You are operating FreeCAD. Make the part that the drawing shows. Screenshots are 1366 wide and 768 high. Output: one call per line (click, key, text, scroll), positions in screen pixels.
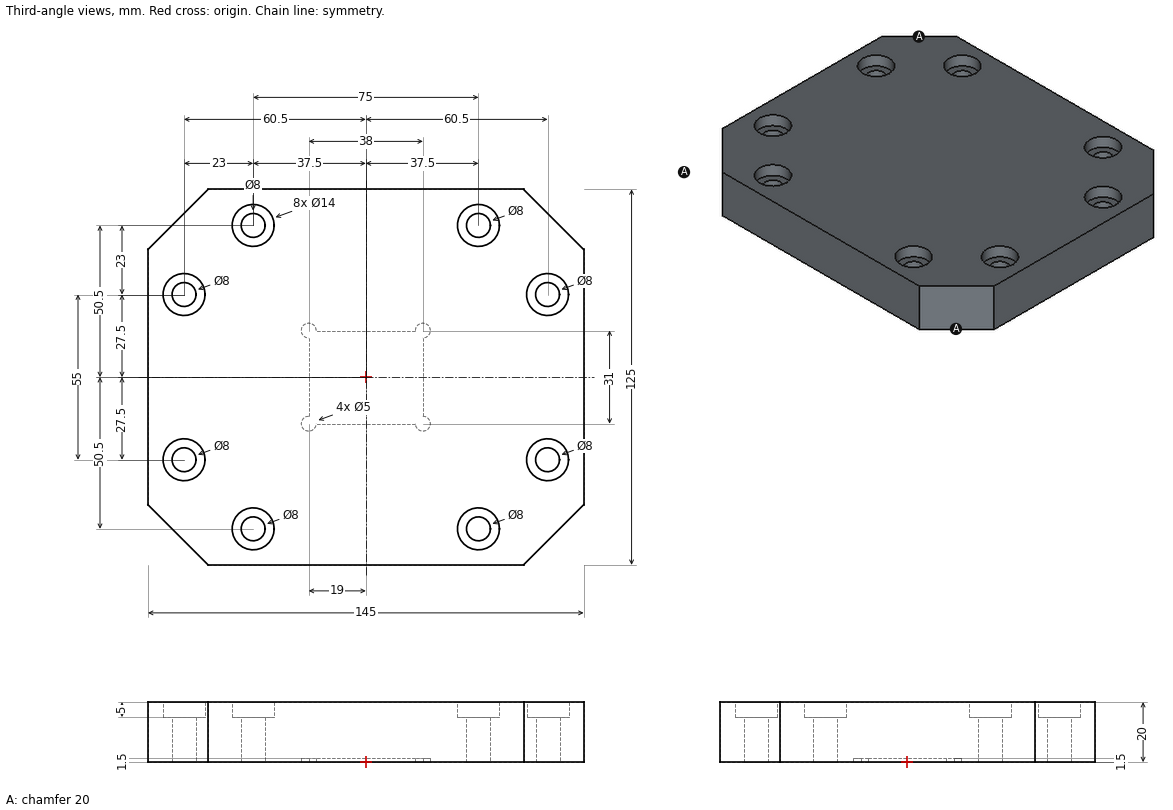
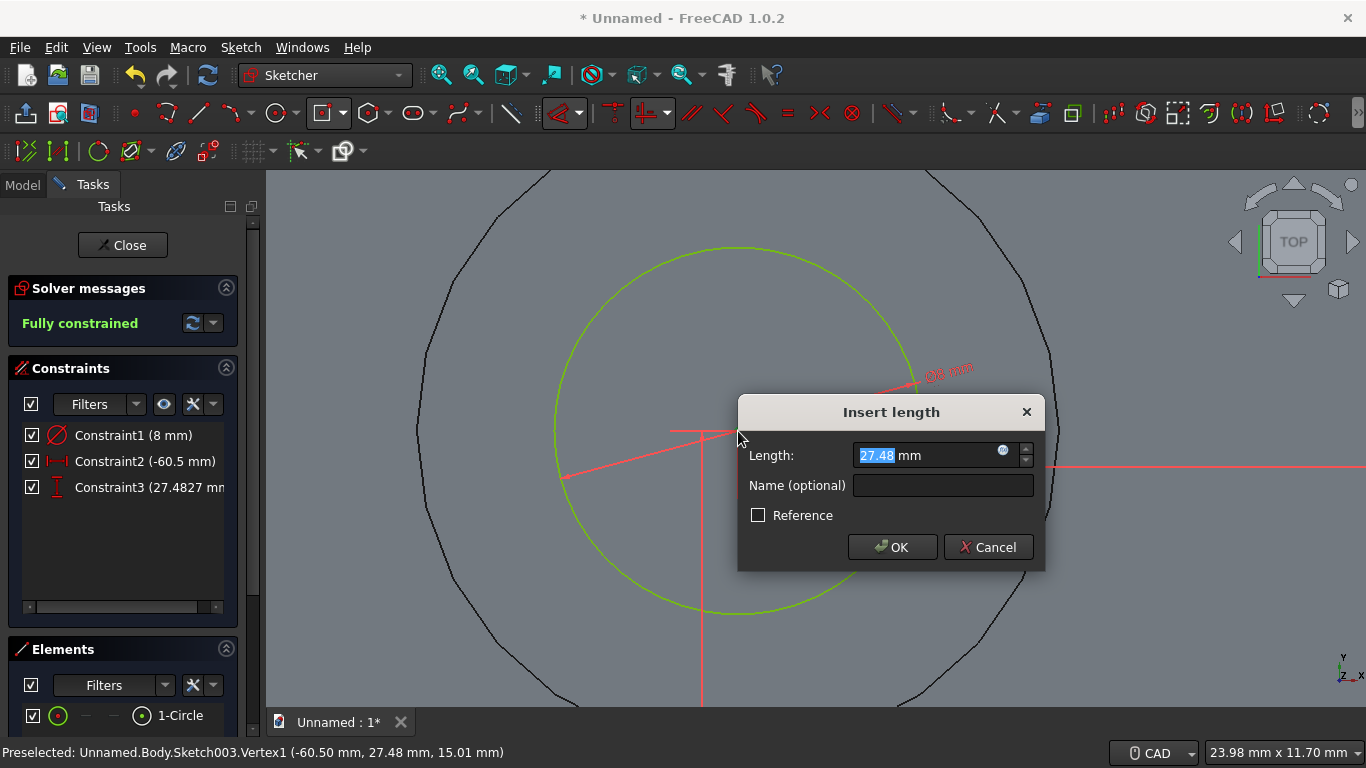
text(27.5)
key(Return)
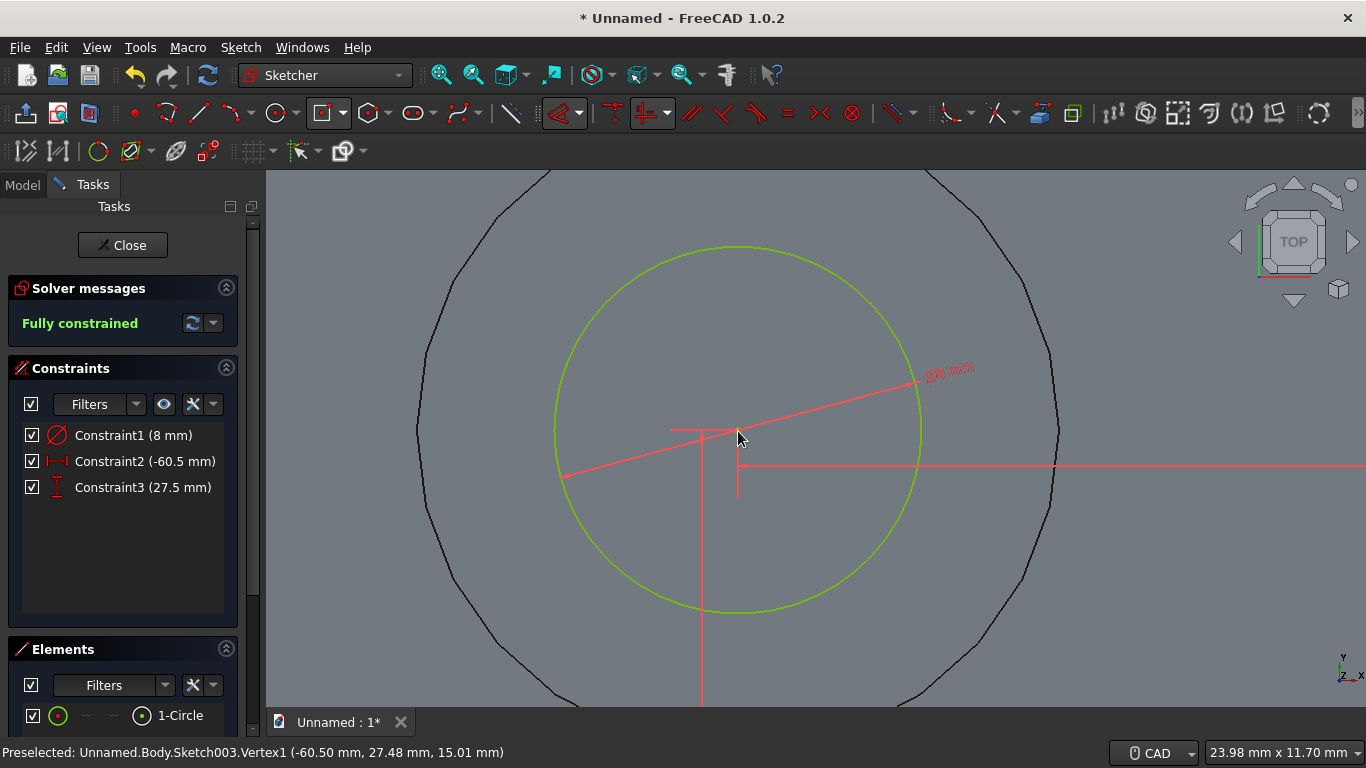
click(123, 245)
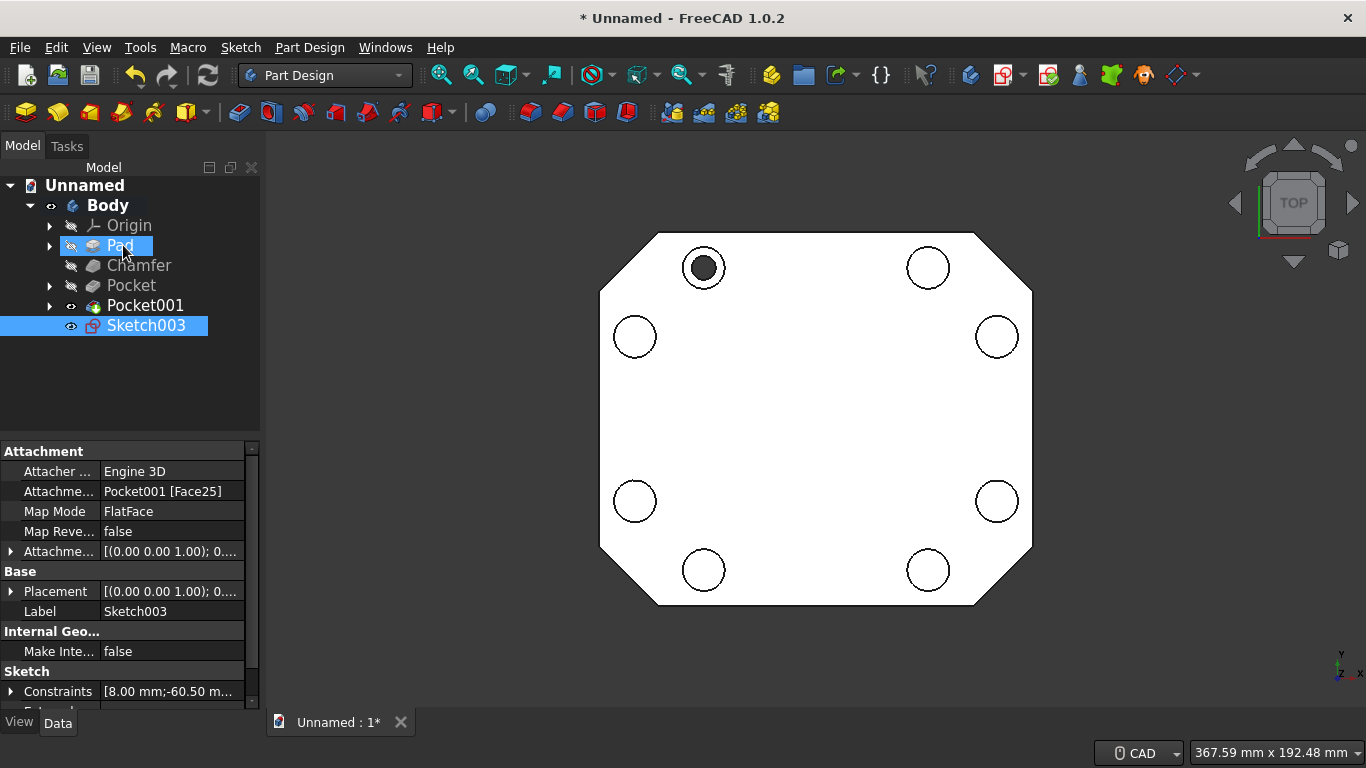
click(240, 112)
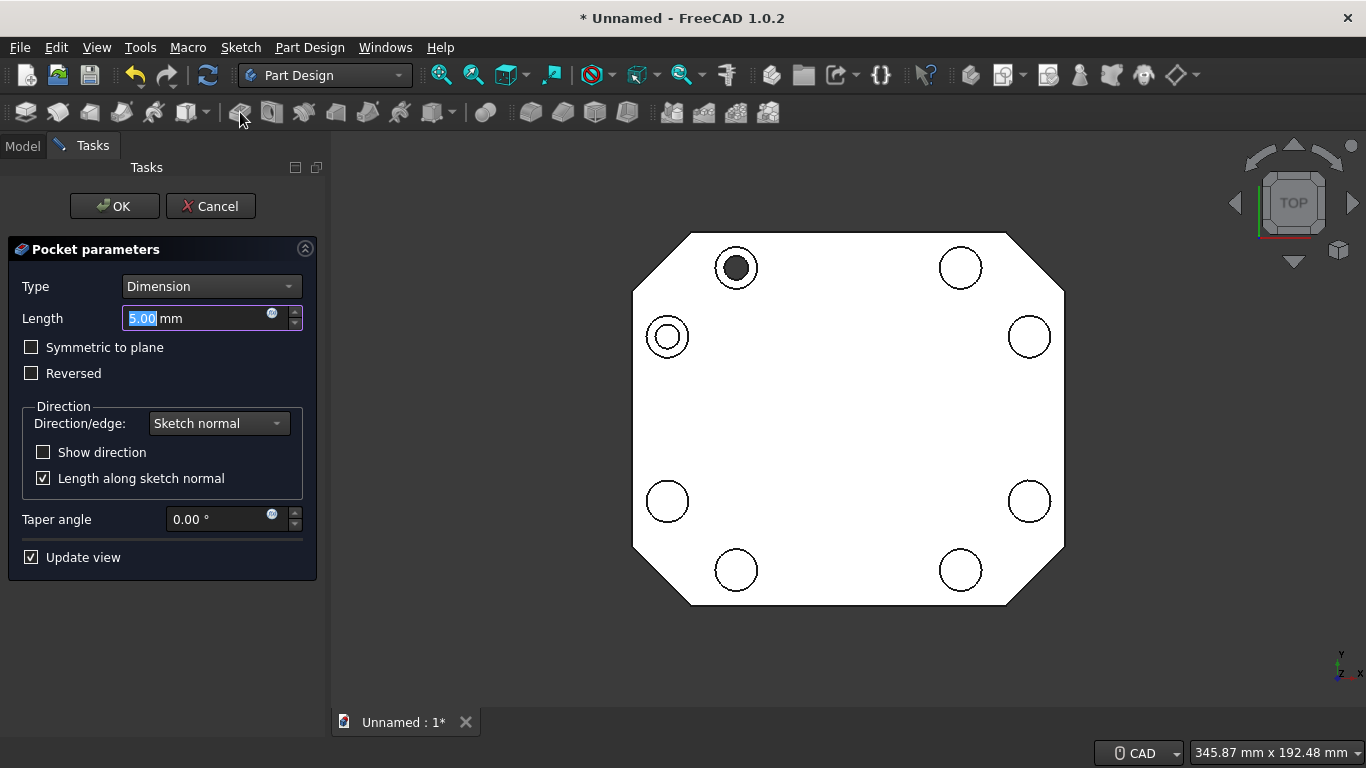
click(212, 286)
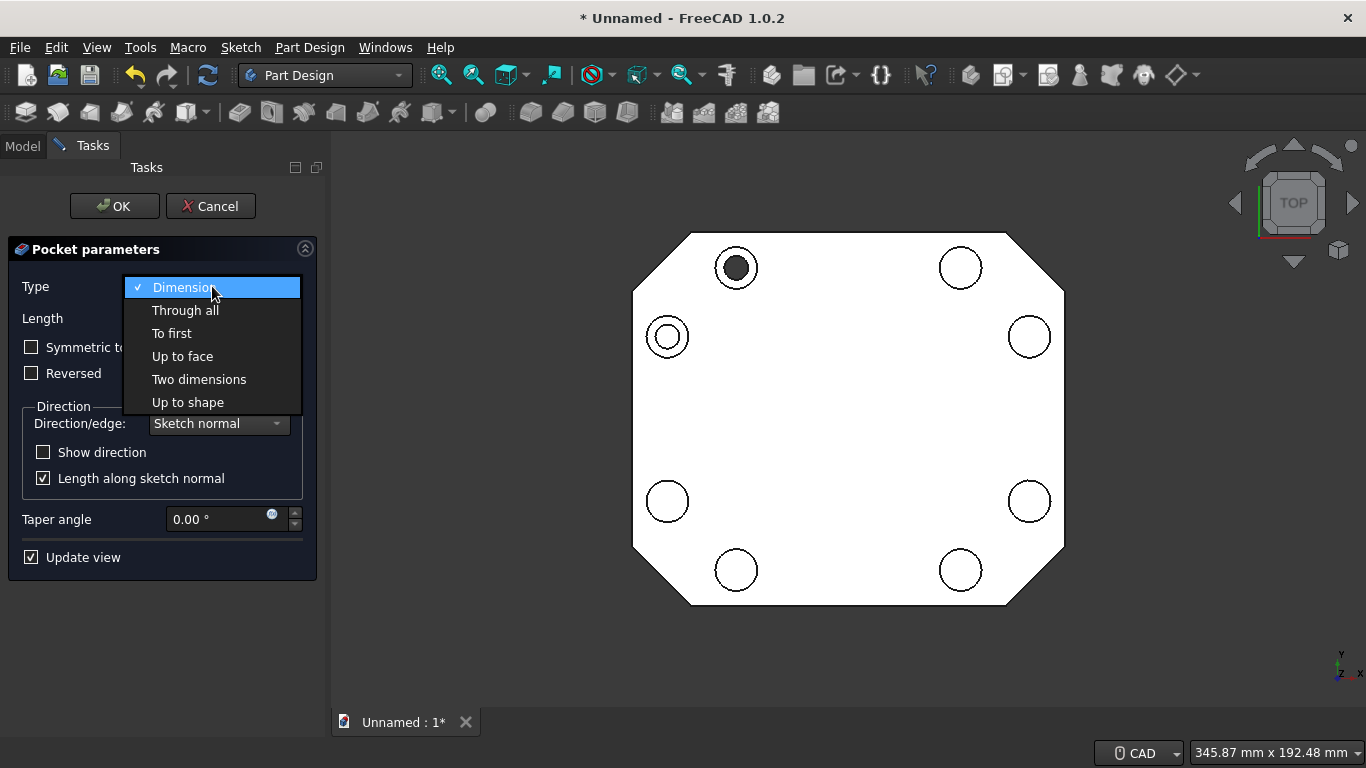
click(212, 334)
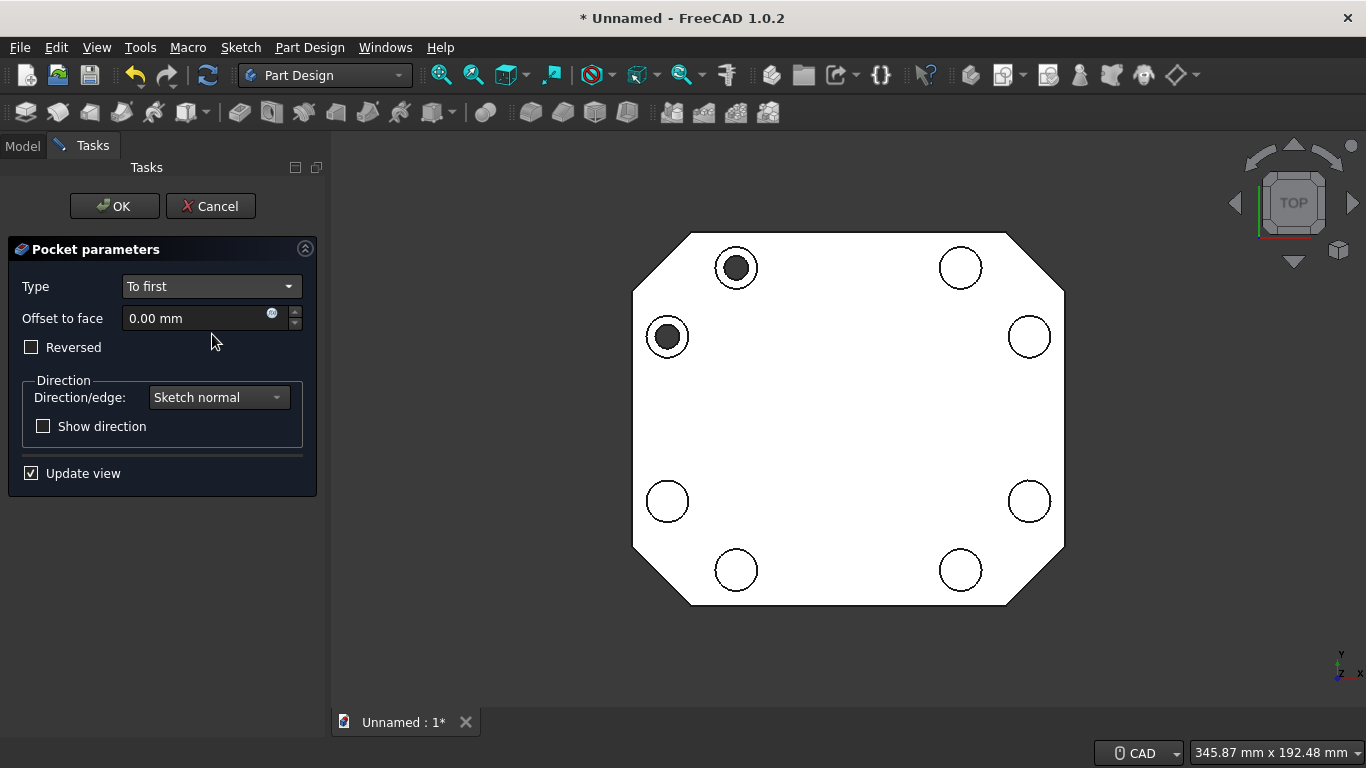
click(115, 206)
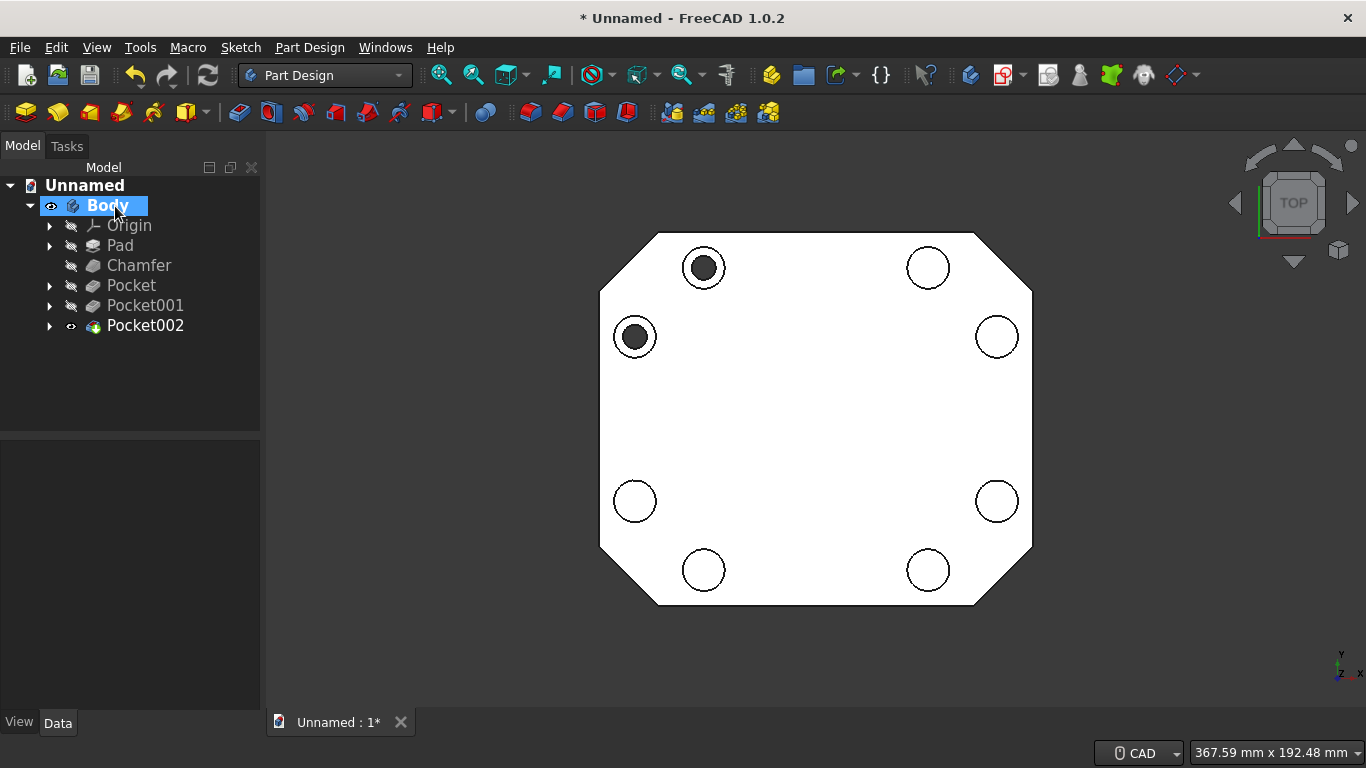
click(635, 500)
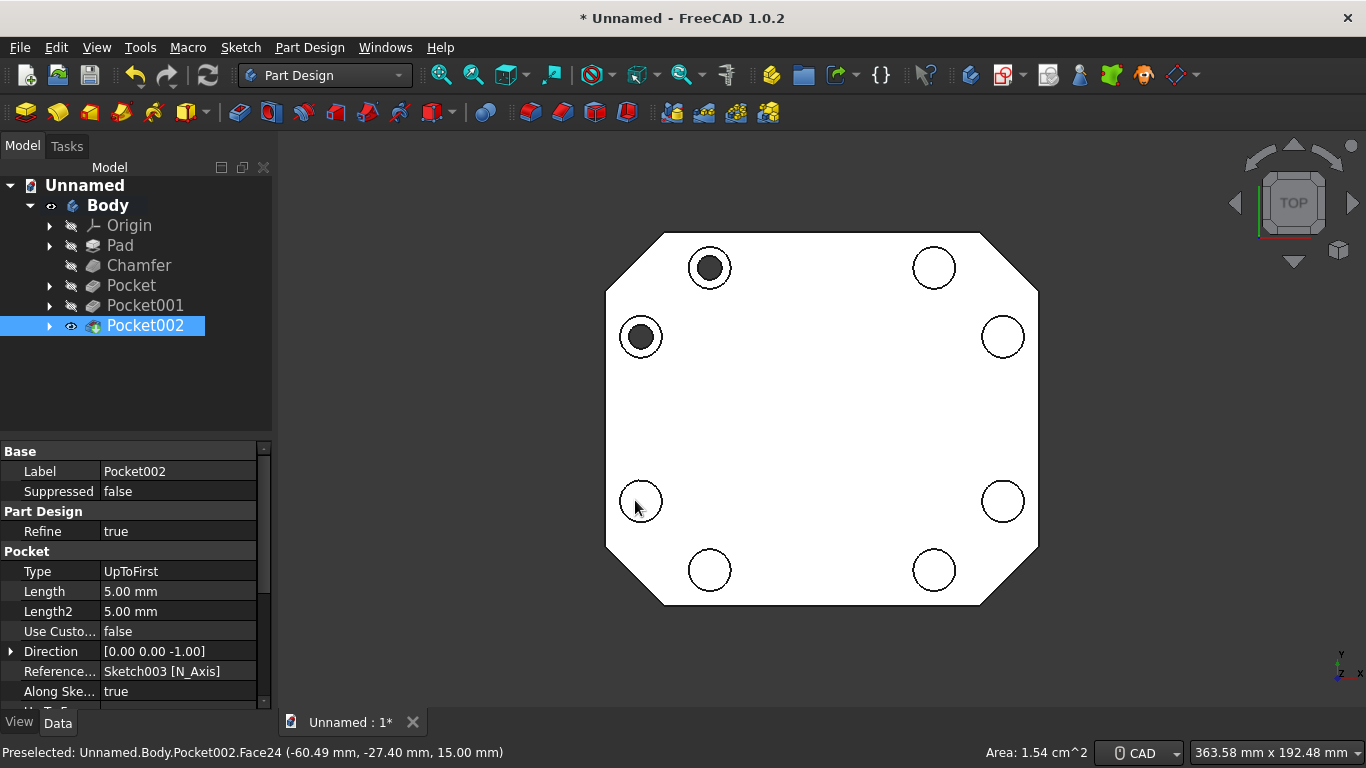
click(1004, 76)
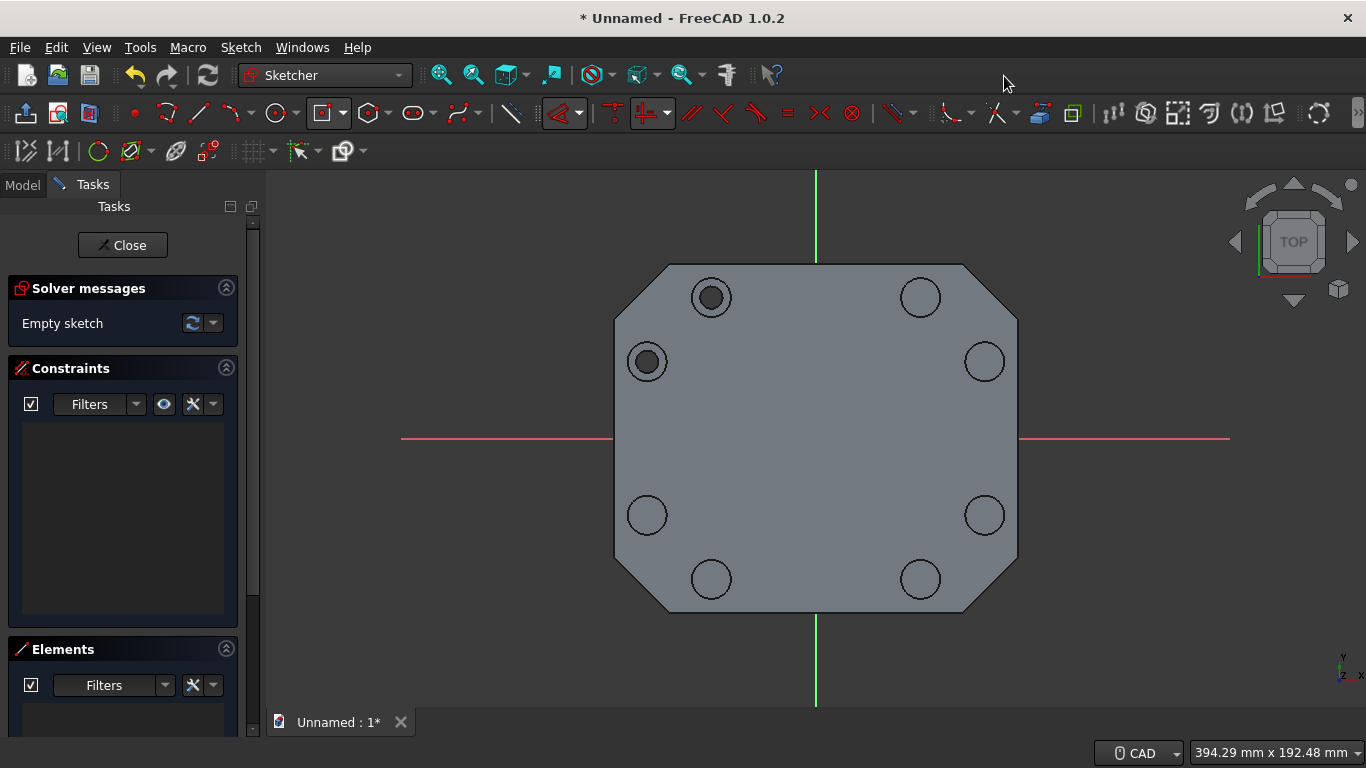
key(q)
key(s)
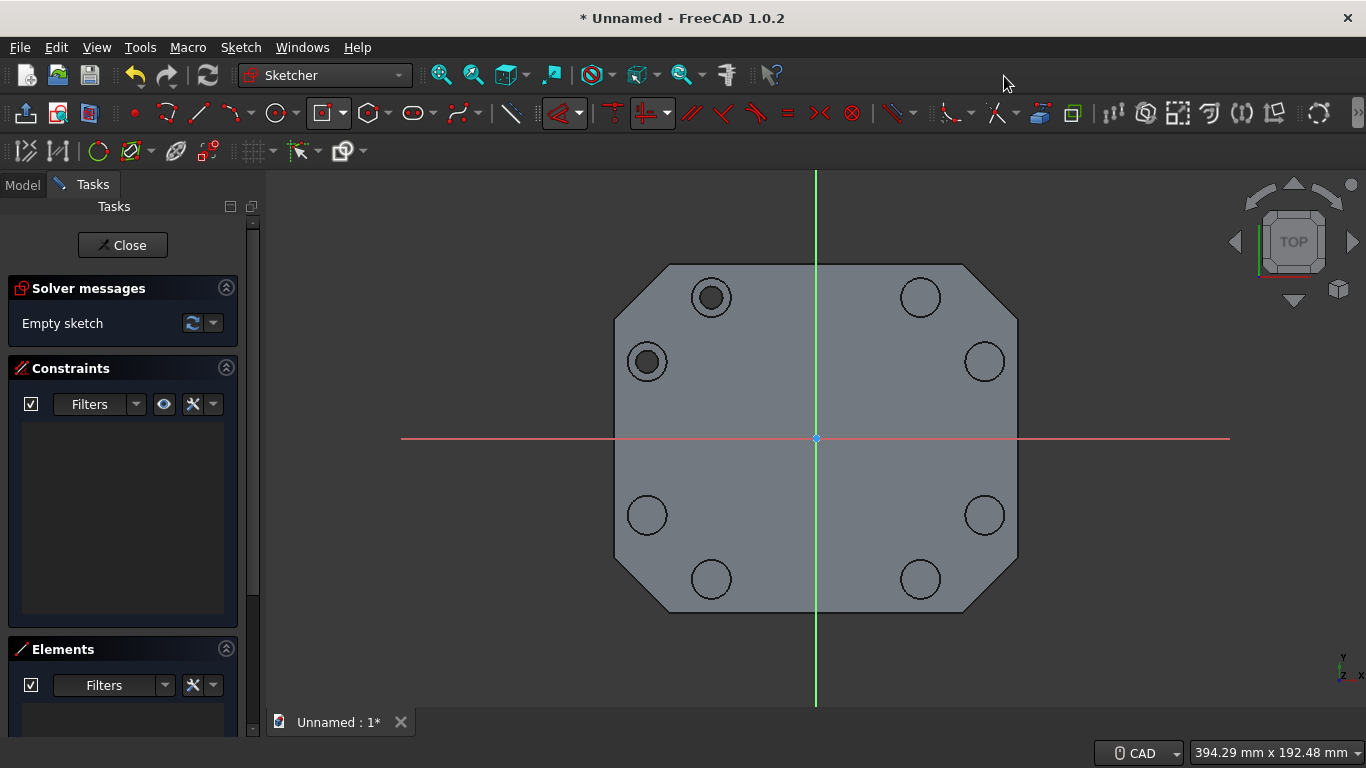
scroll(641, 520, up, 14)